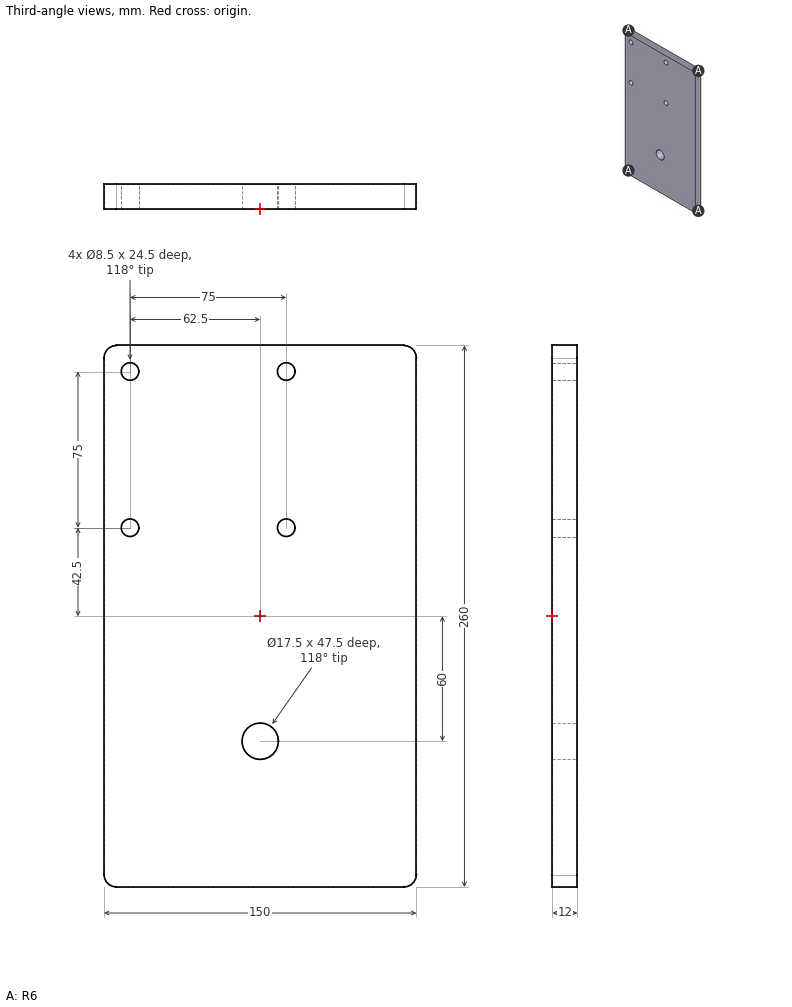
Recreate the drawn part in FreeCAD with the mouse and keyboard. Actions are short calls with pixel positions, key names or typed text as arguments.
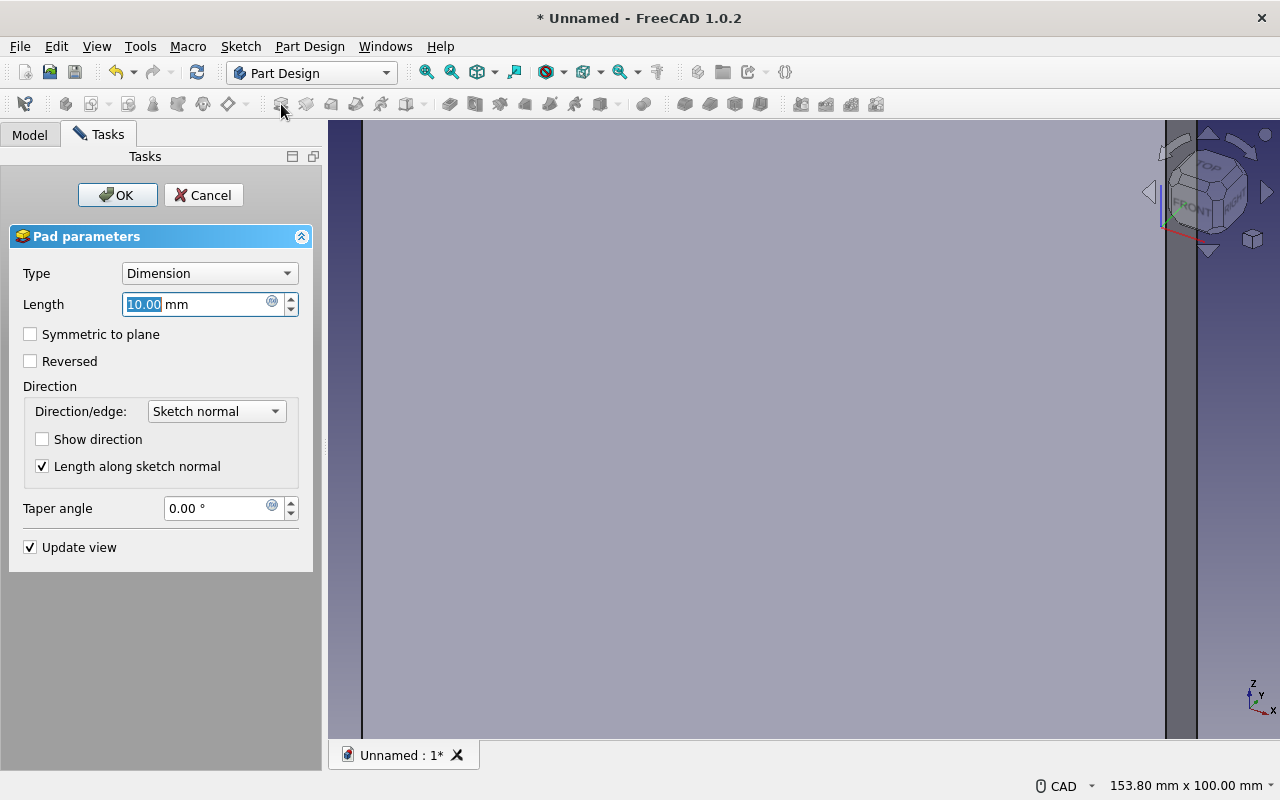
text(12)
key(Tab)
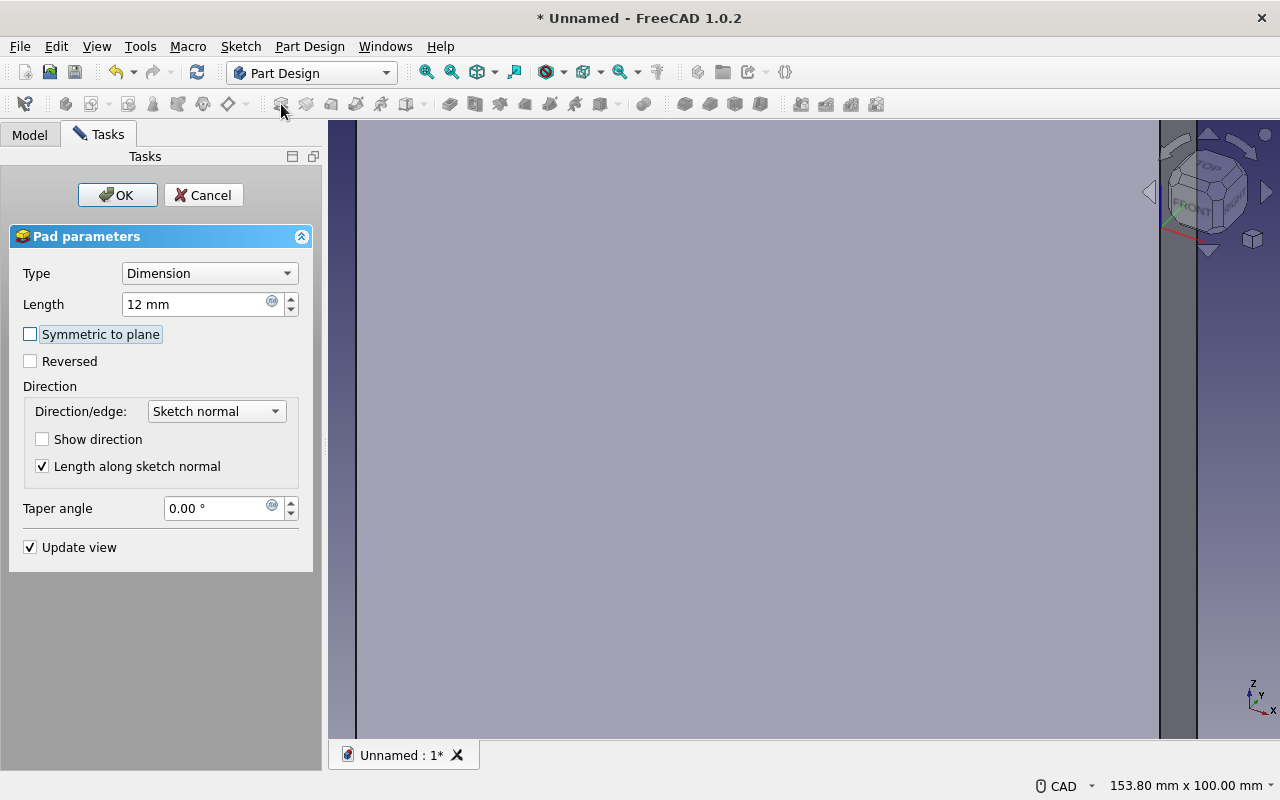
click(31, 361)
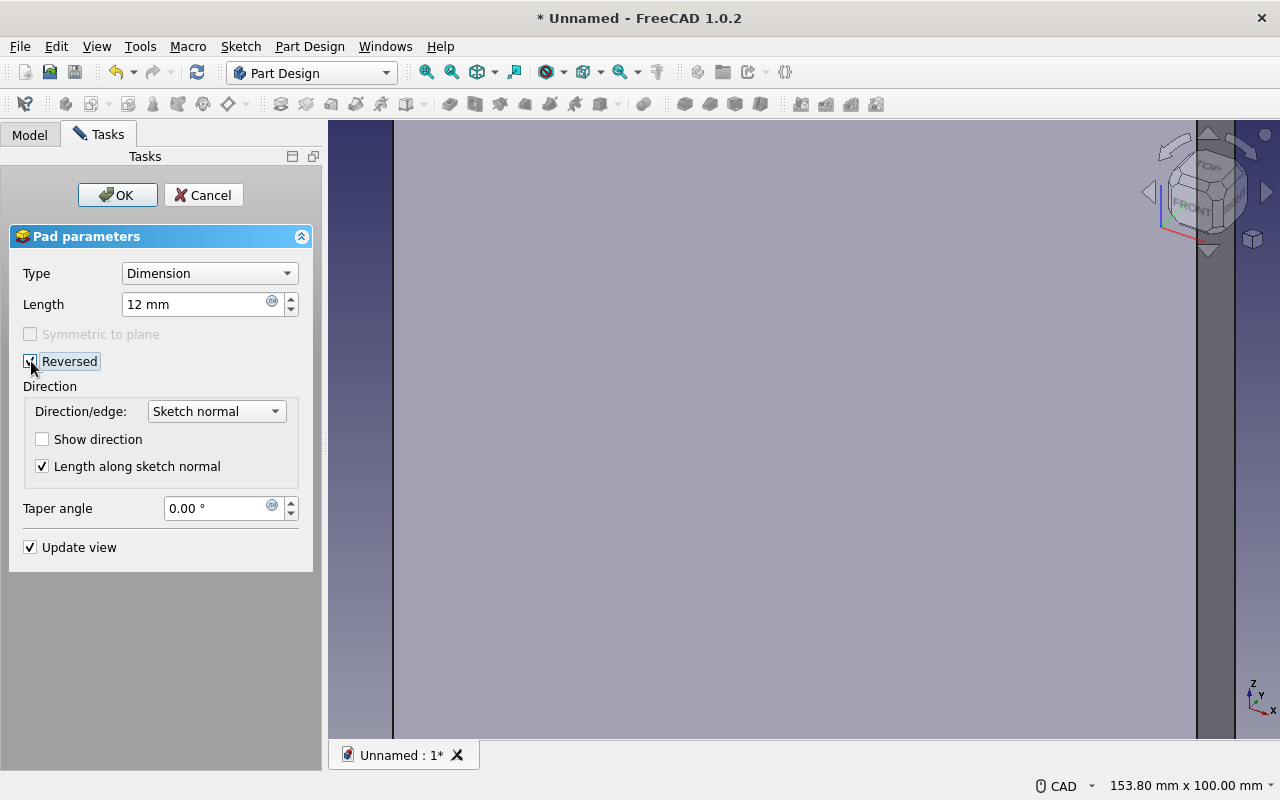
click(118, 195)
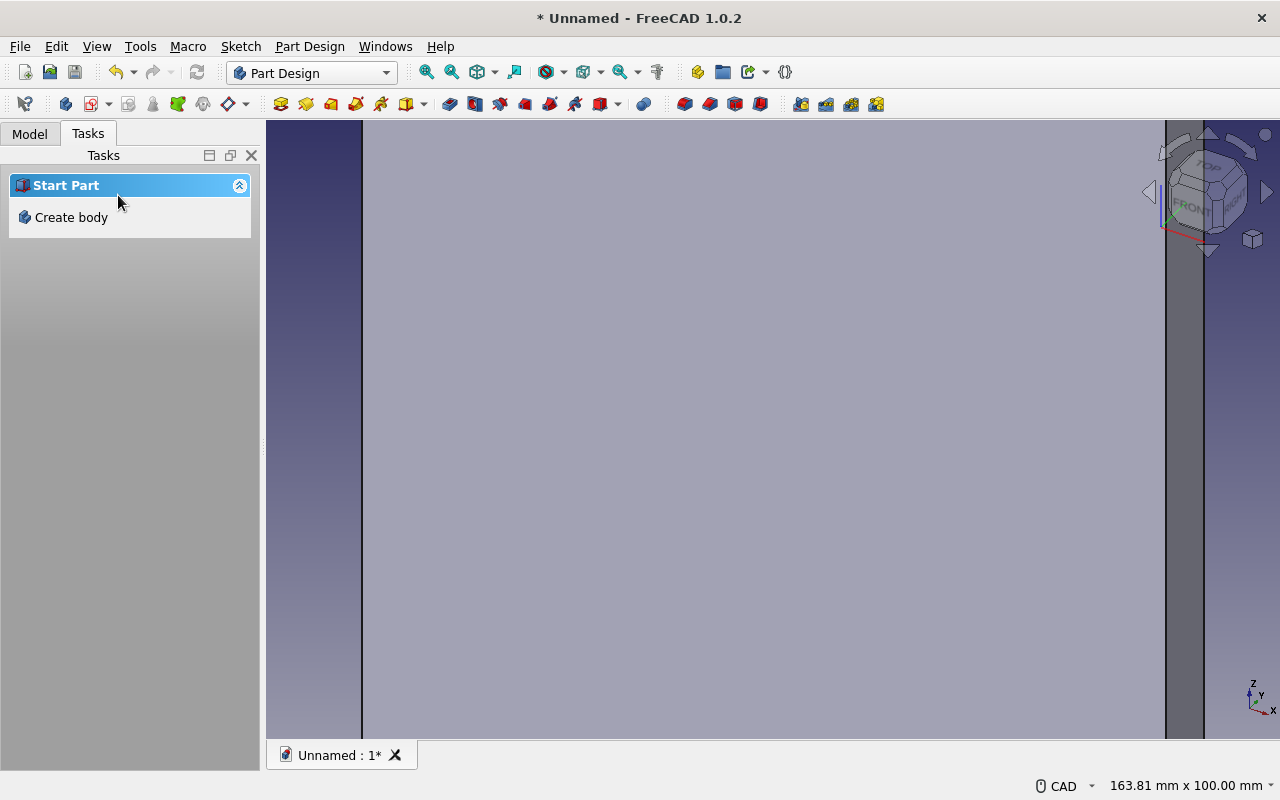
key(v)
key(f)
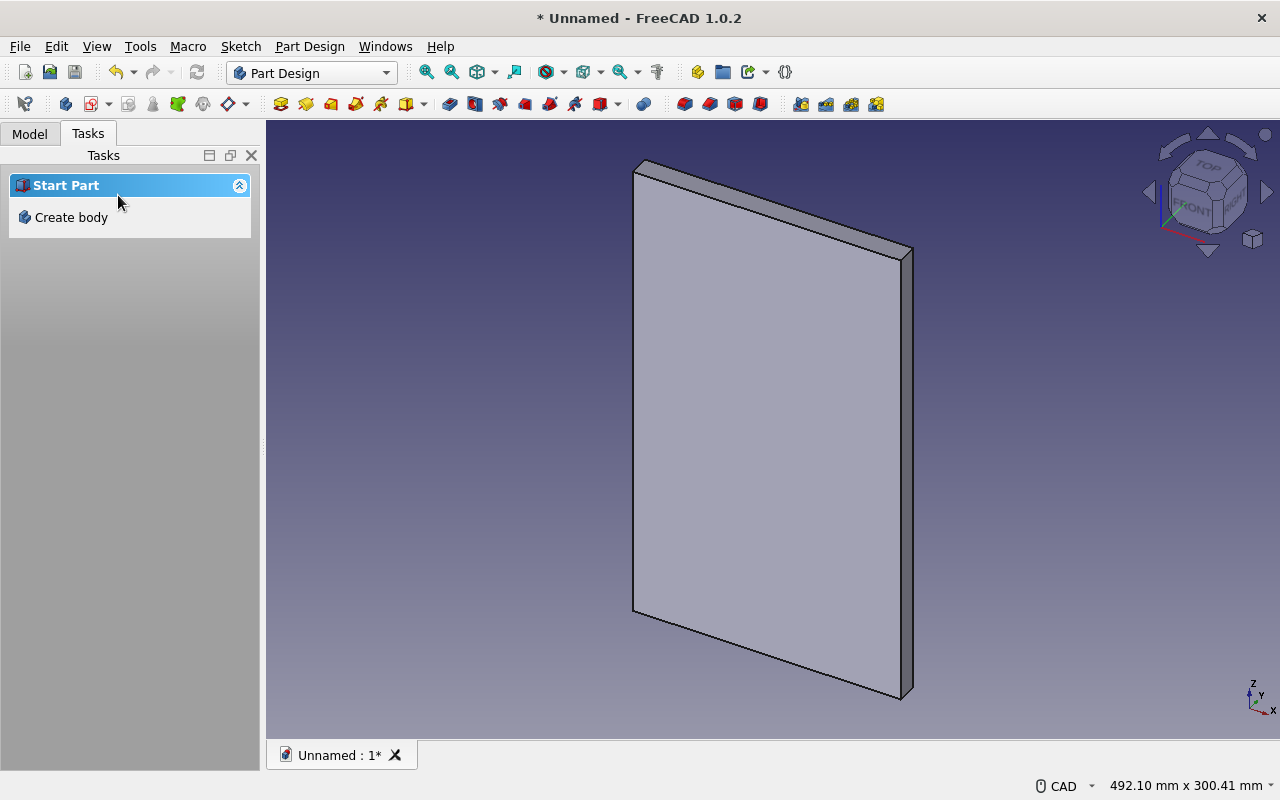
click(907, 253)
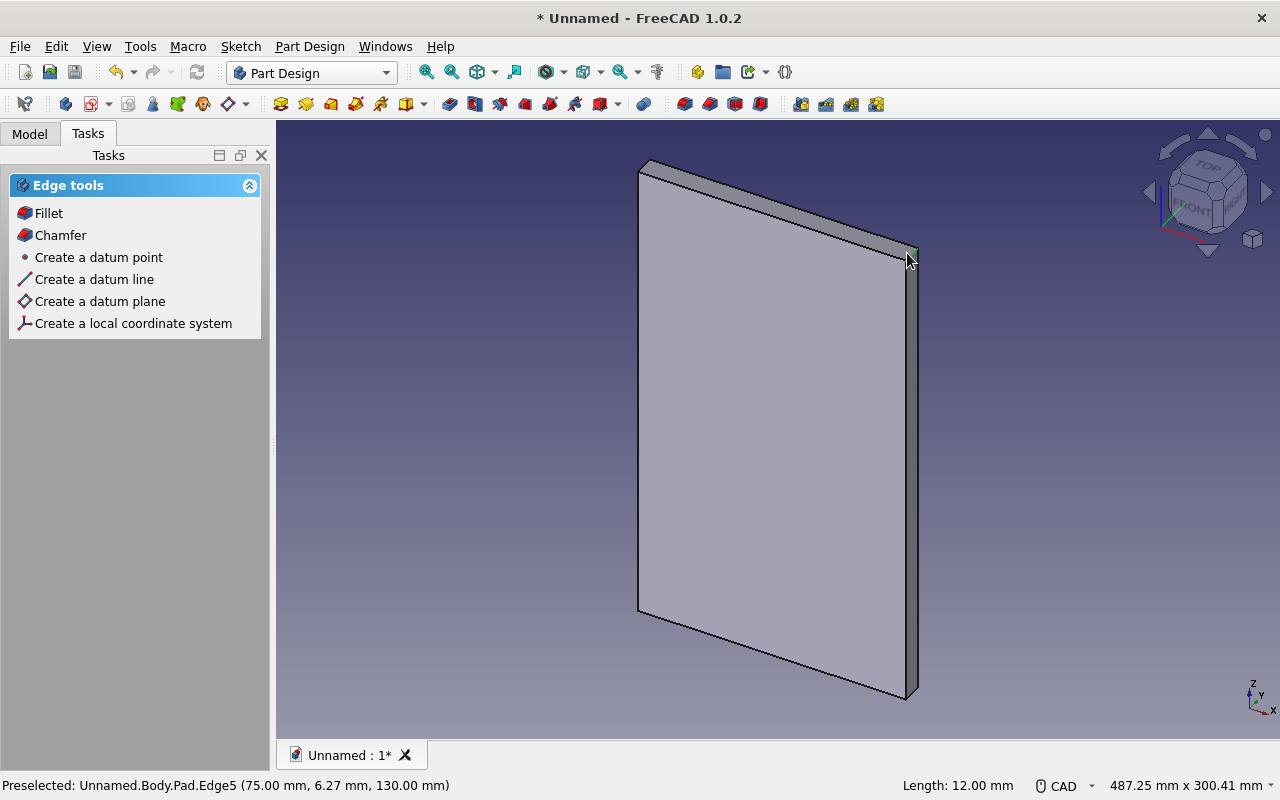
key(0)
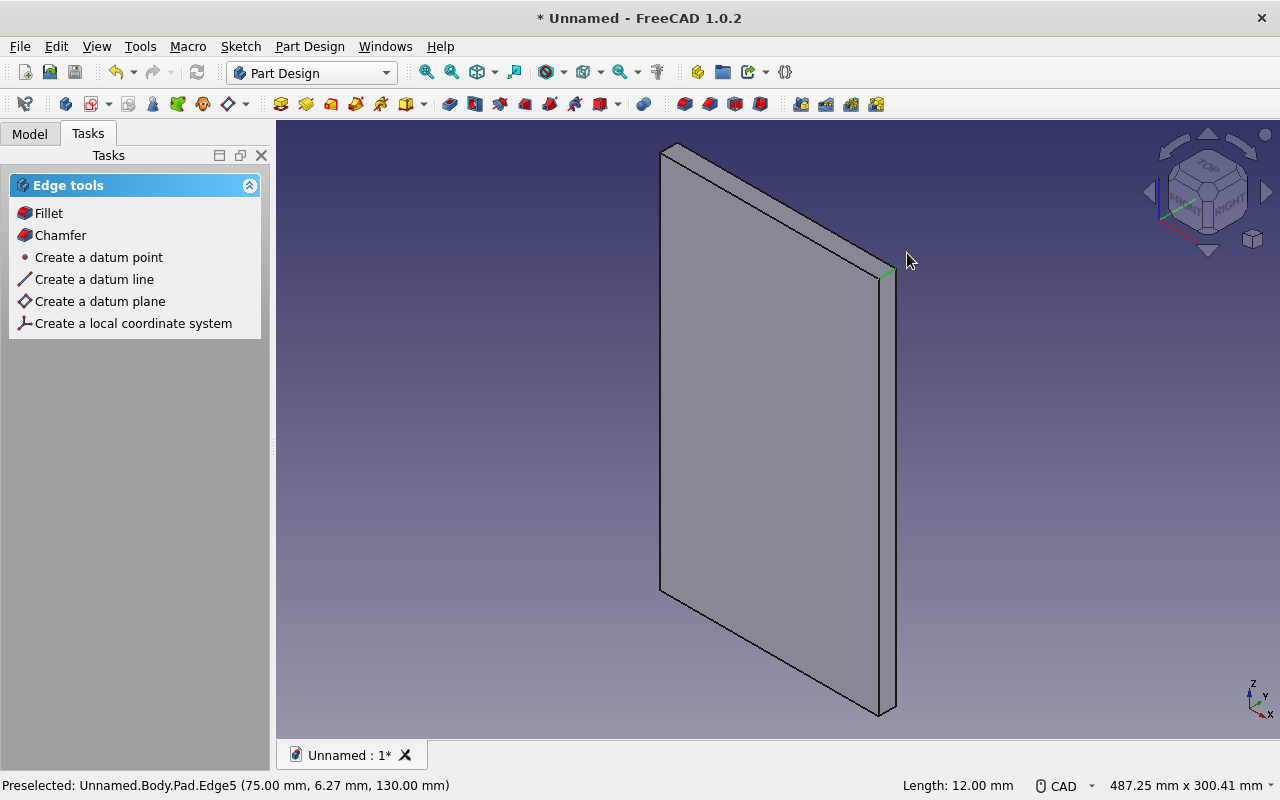
key(2)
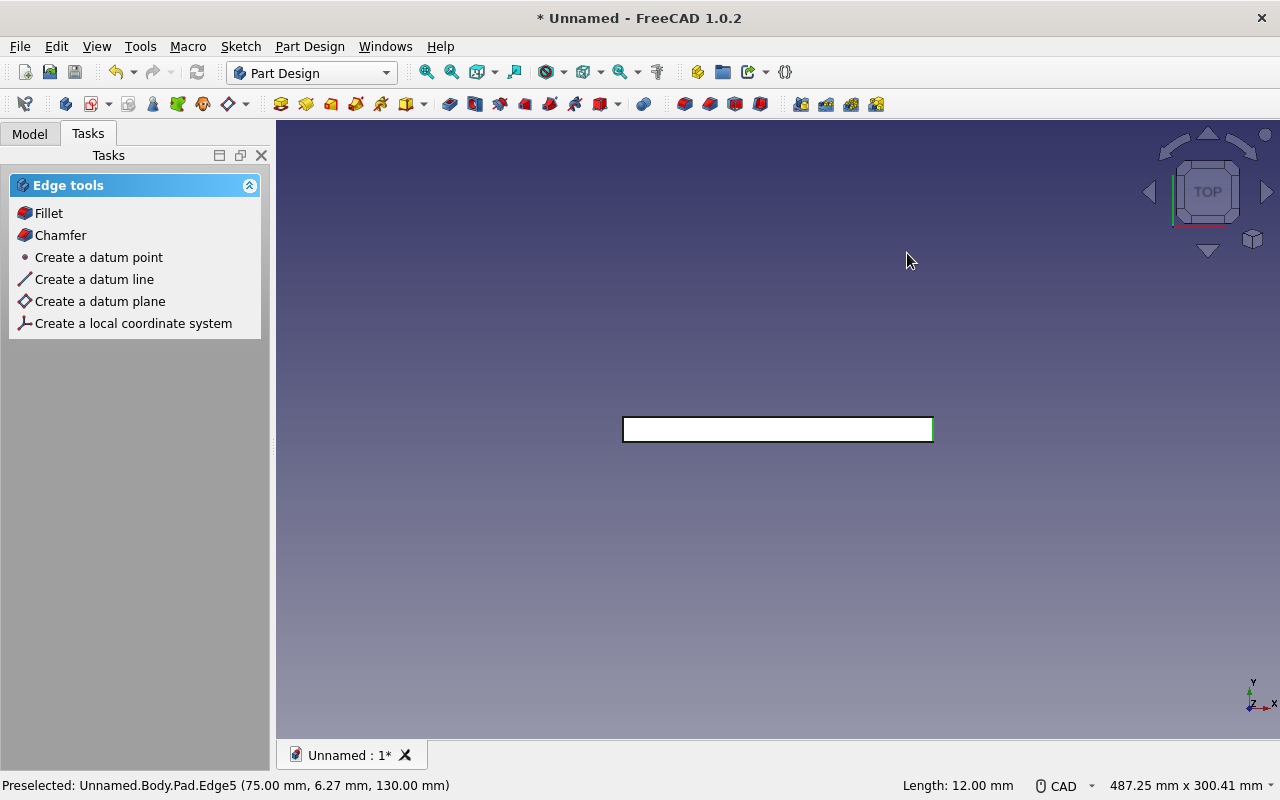
key(v)
key(f)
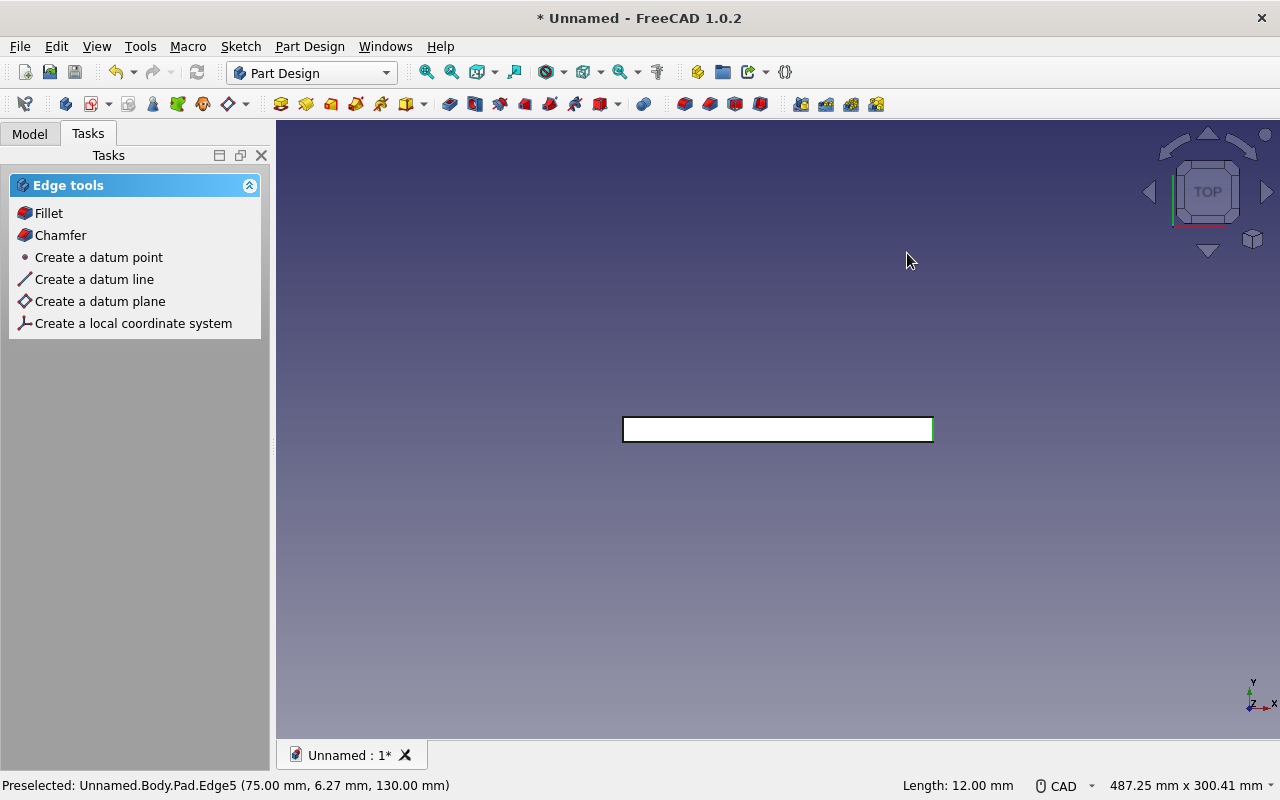
click(623, 428, ctrl)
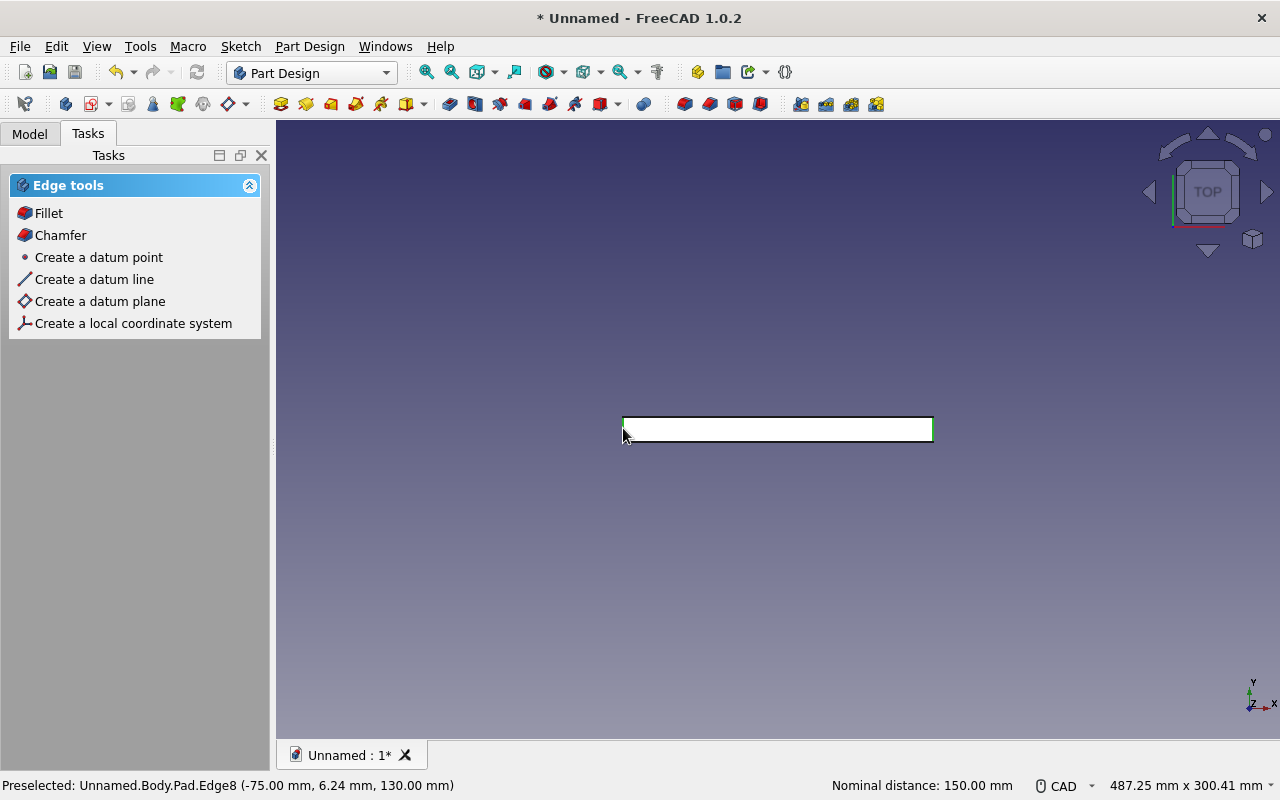
key(1)